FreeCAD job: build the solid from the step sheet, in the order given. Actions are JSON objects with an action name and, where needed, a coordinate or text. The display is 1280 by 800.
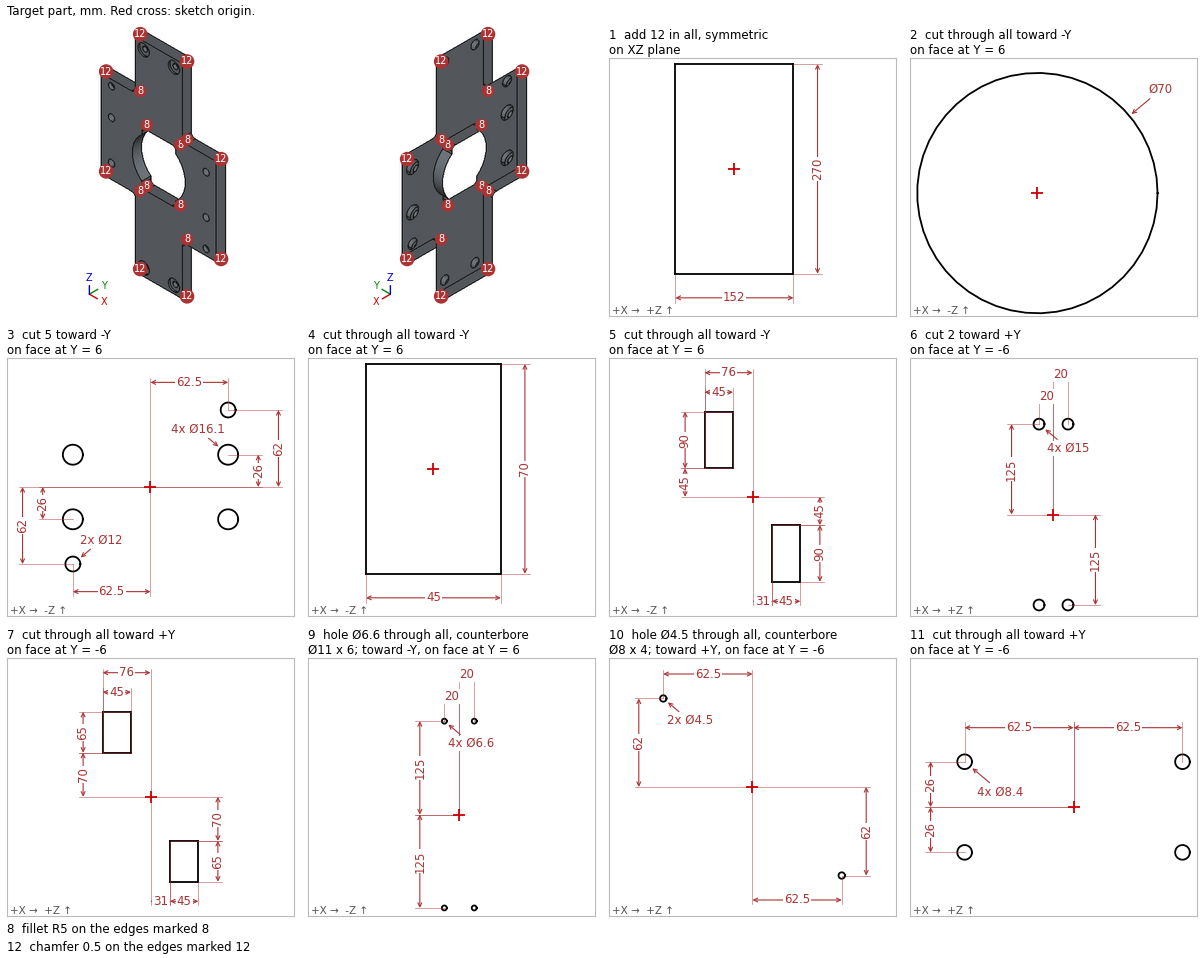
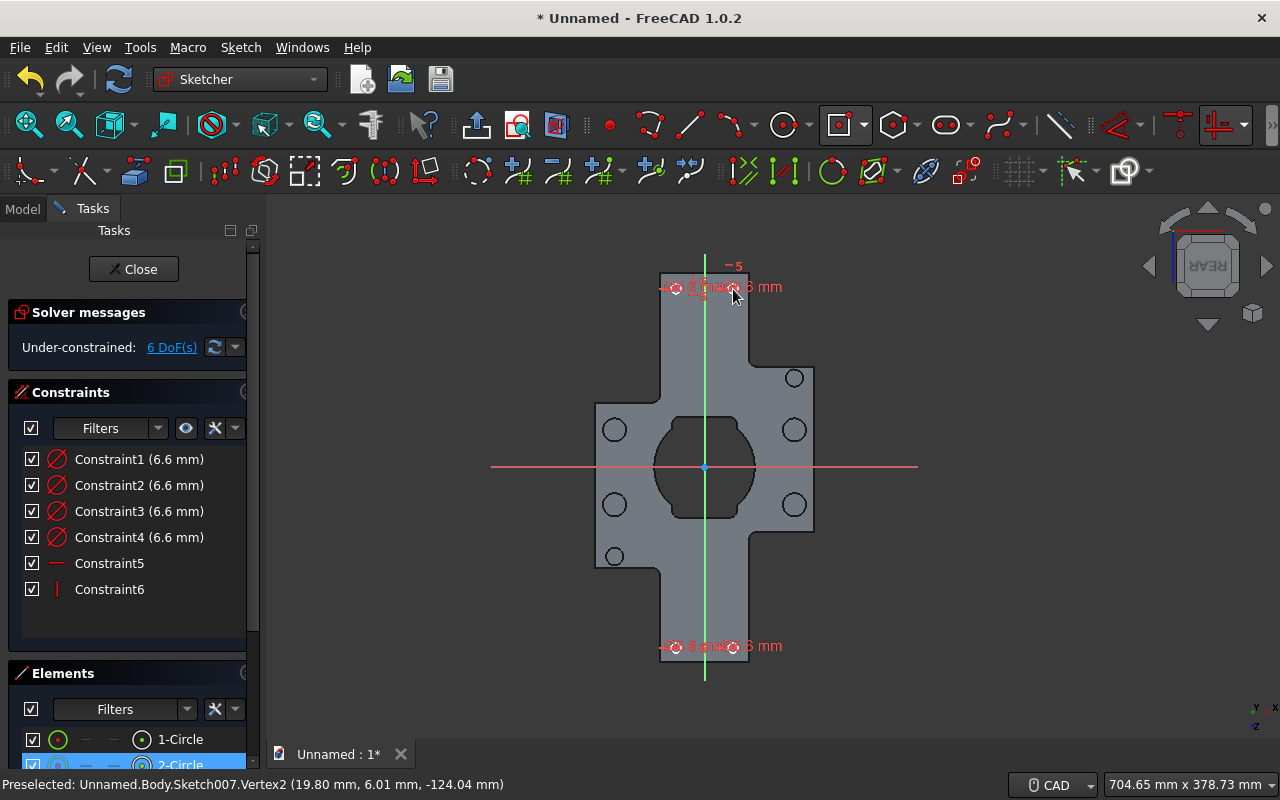
{"action": "left_click", "coordinate": [733, 648]}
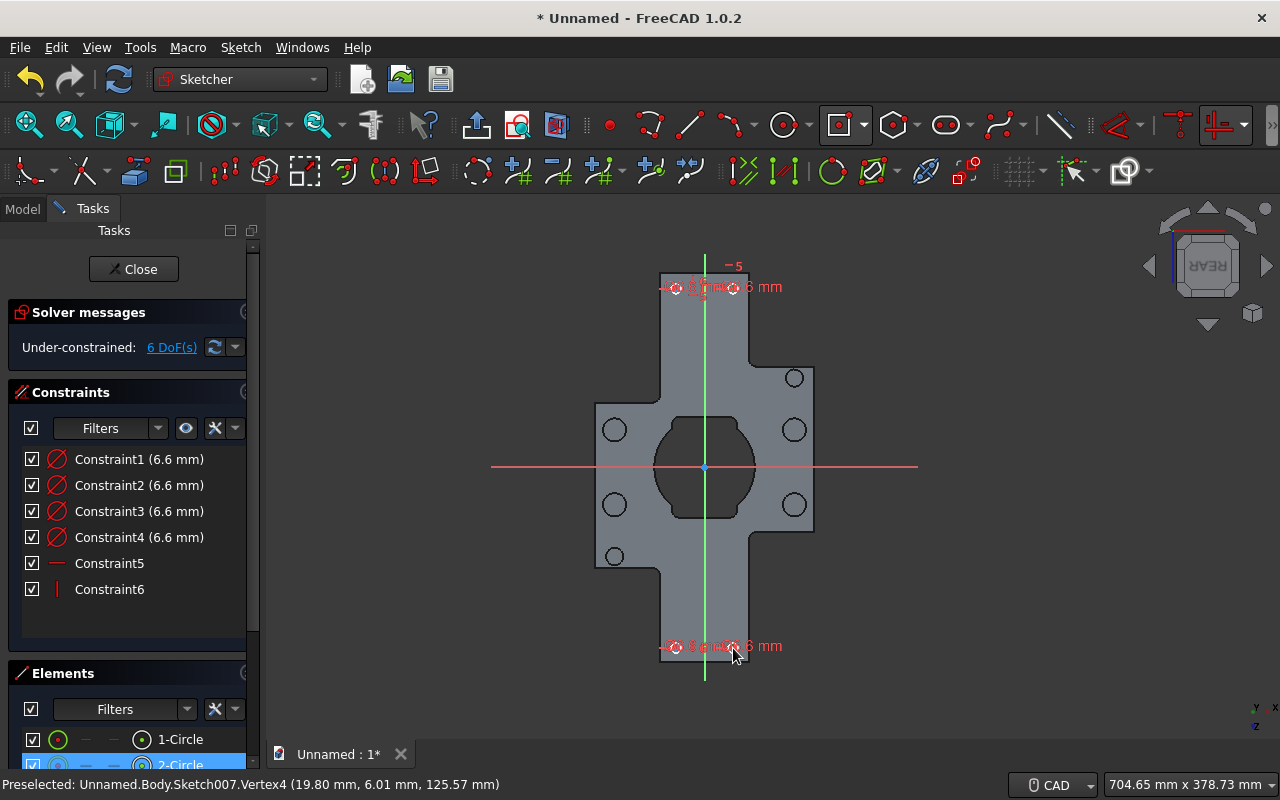
{"action": "key", "text": "v"}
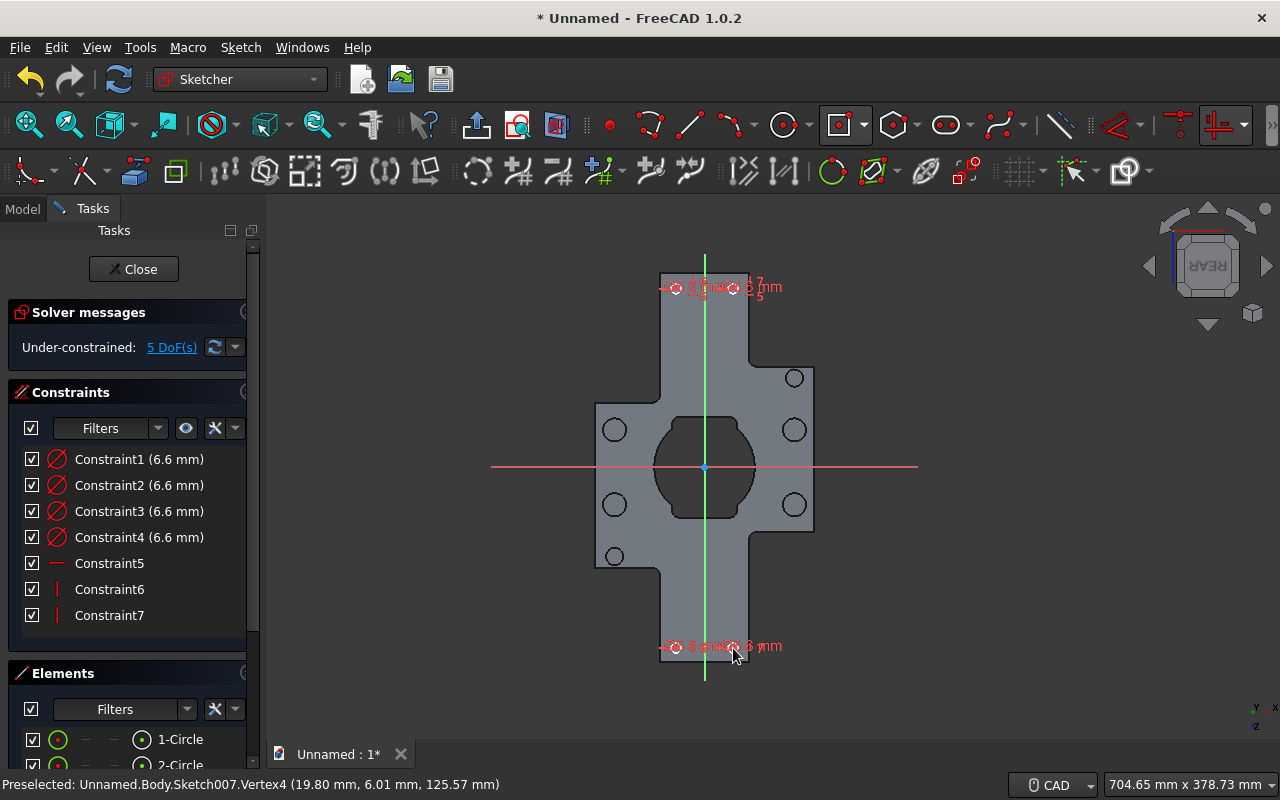
{"action": "left_click", "coordinate": [676, 648]}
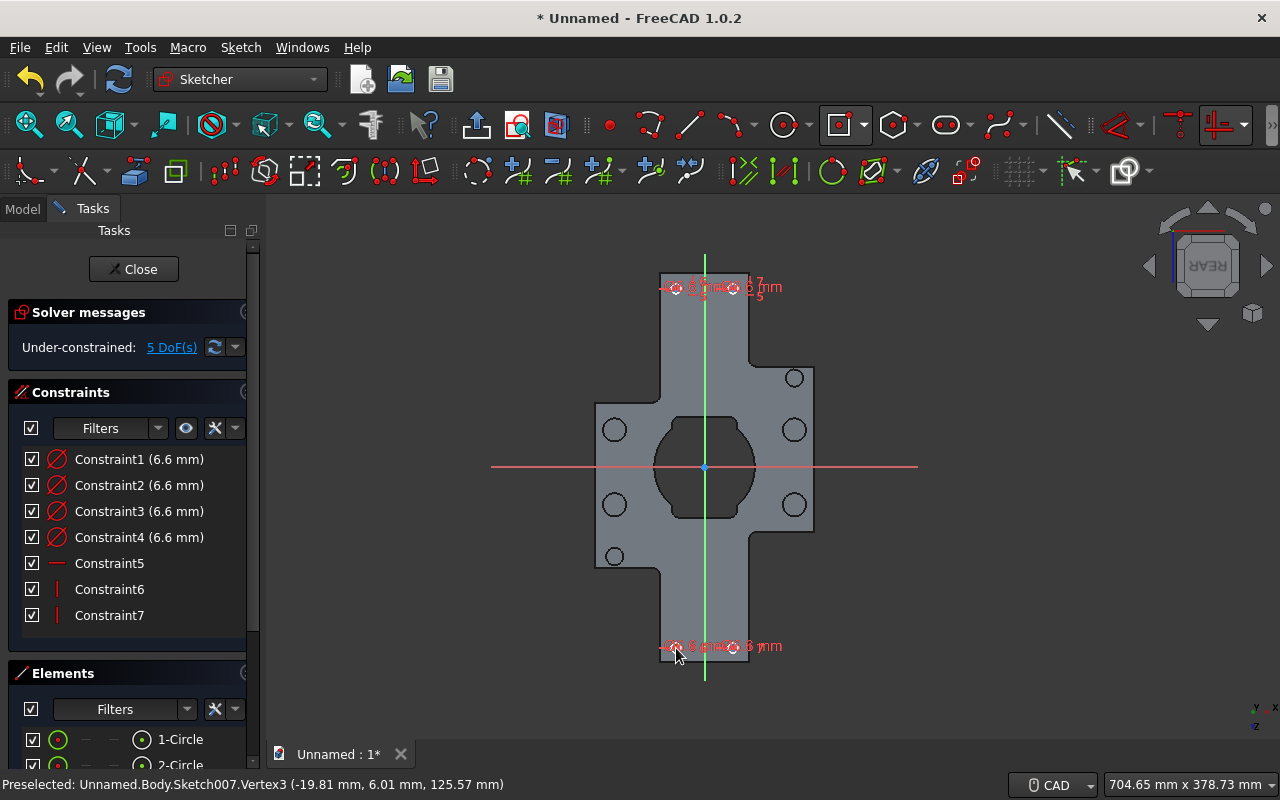
{"action": "left_click", "coordinate": [733, 648]}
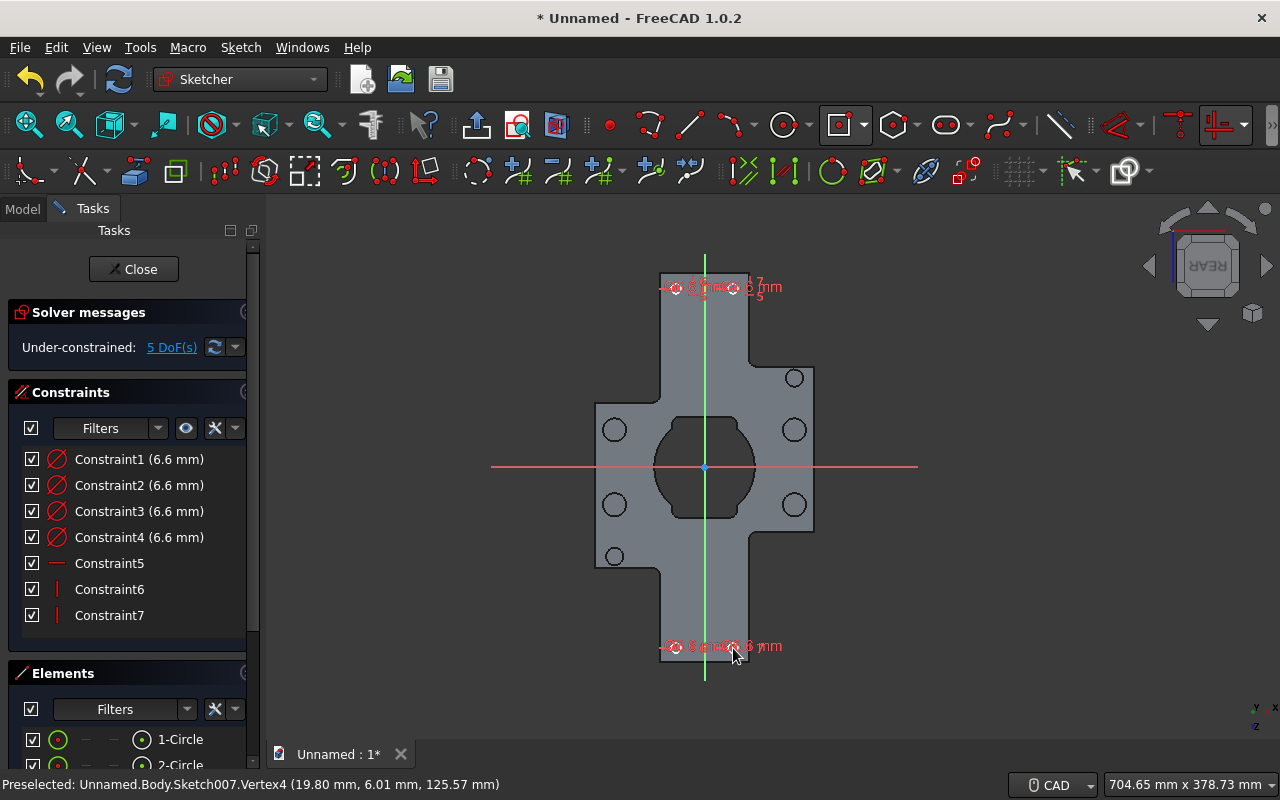
{"action": "key", "text": "h"}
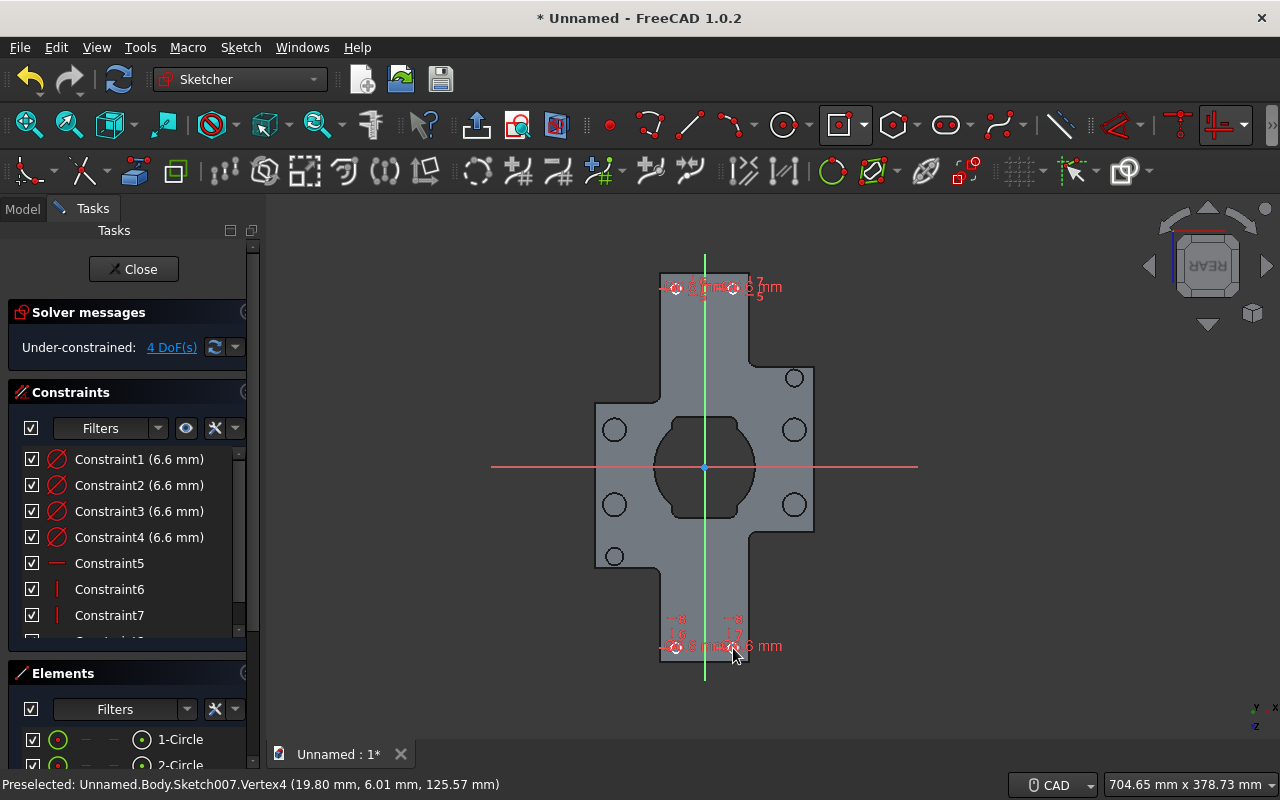
{"action": "key", "text": "d"}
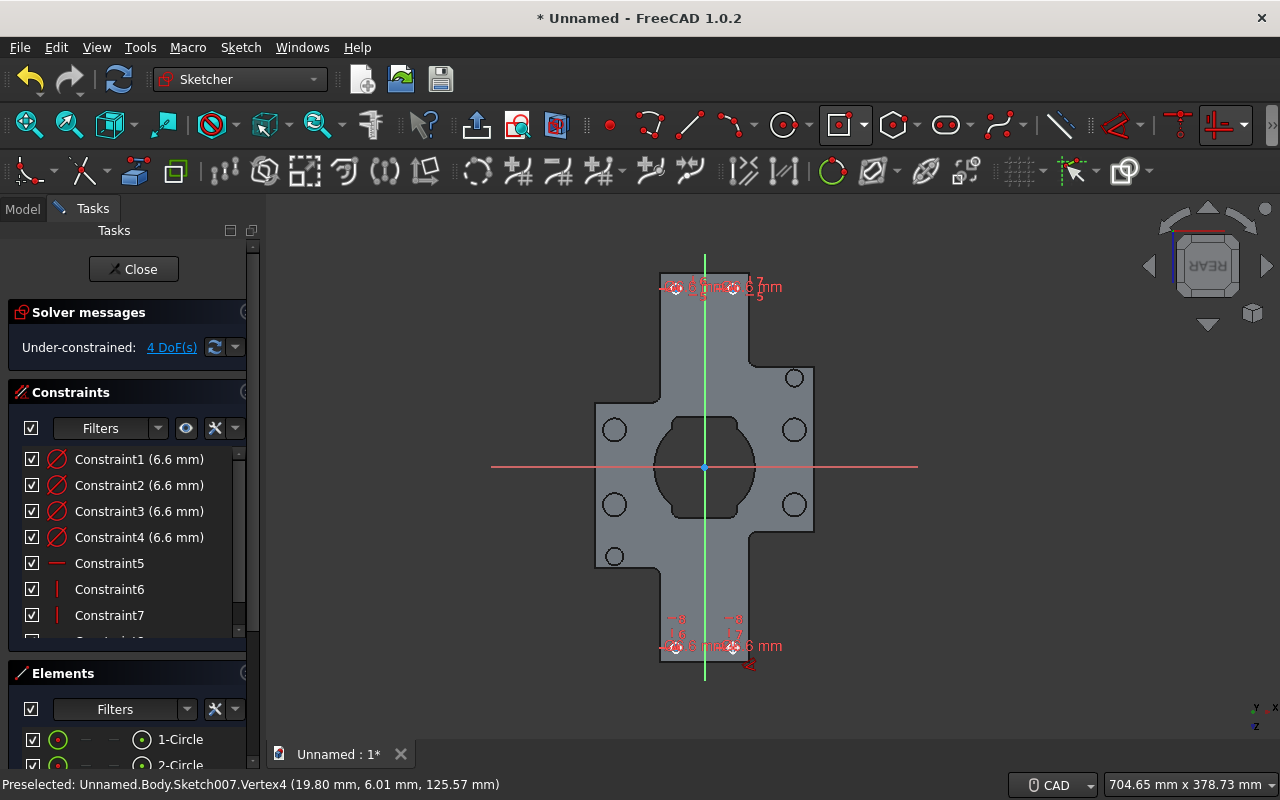
{"action": "scroll", "coordinate": [676, 289], "scroll_direction": "up", "scroll_amount": 2}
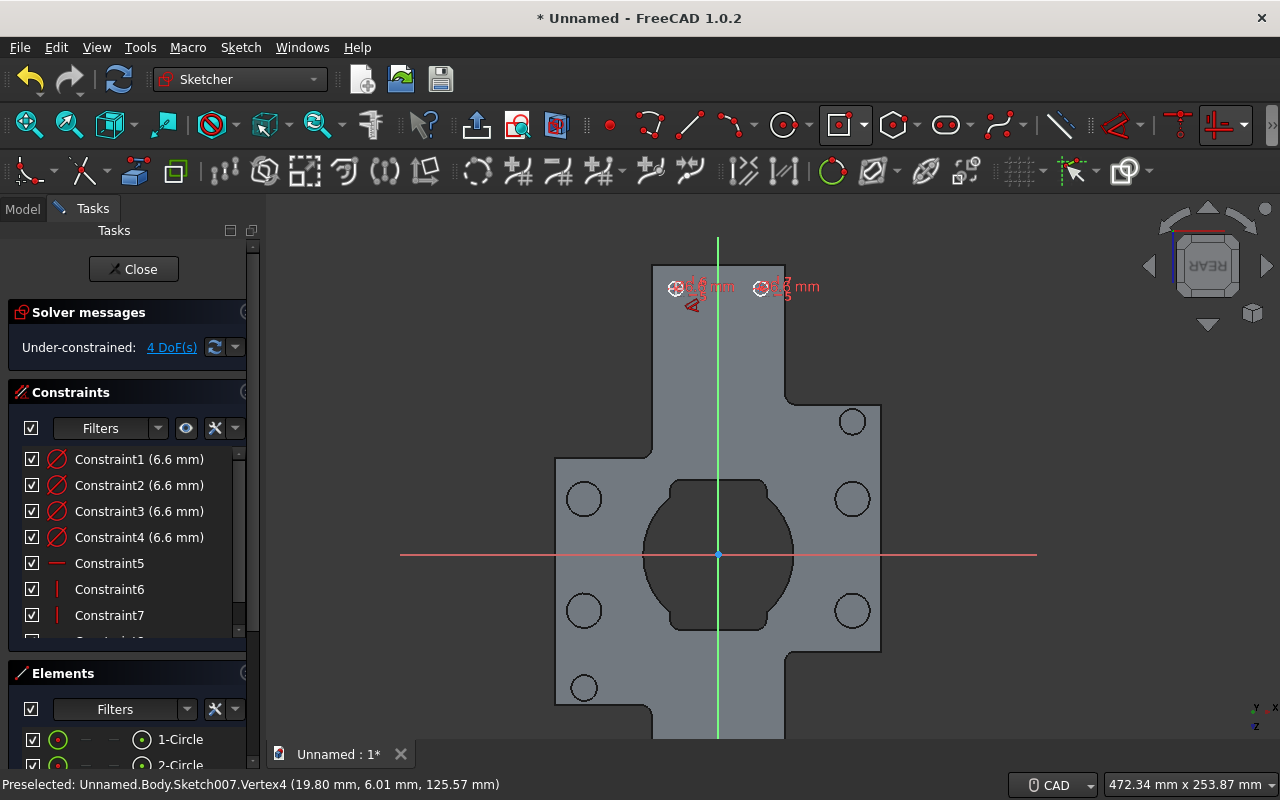
{"action": "left_click", "coordinate": [676, 289]}
{"action": "left_click", "coordinate": [697, 255]}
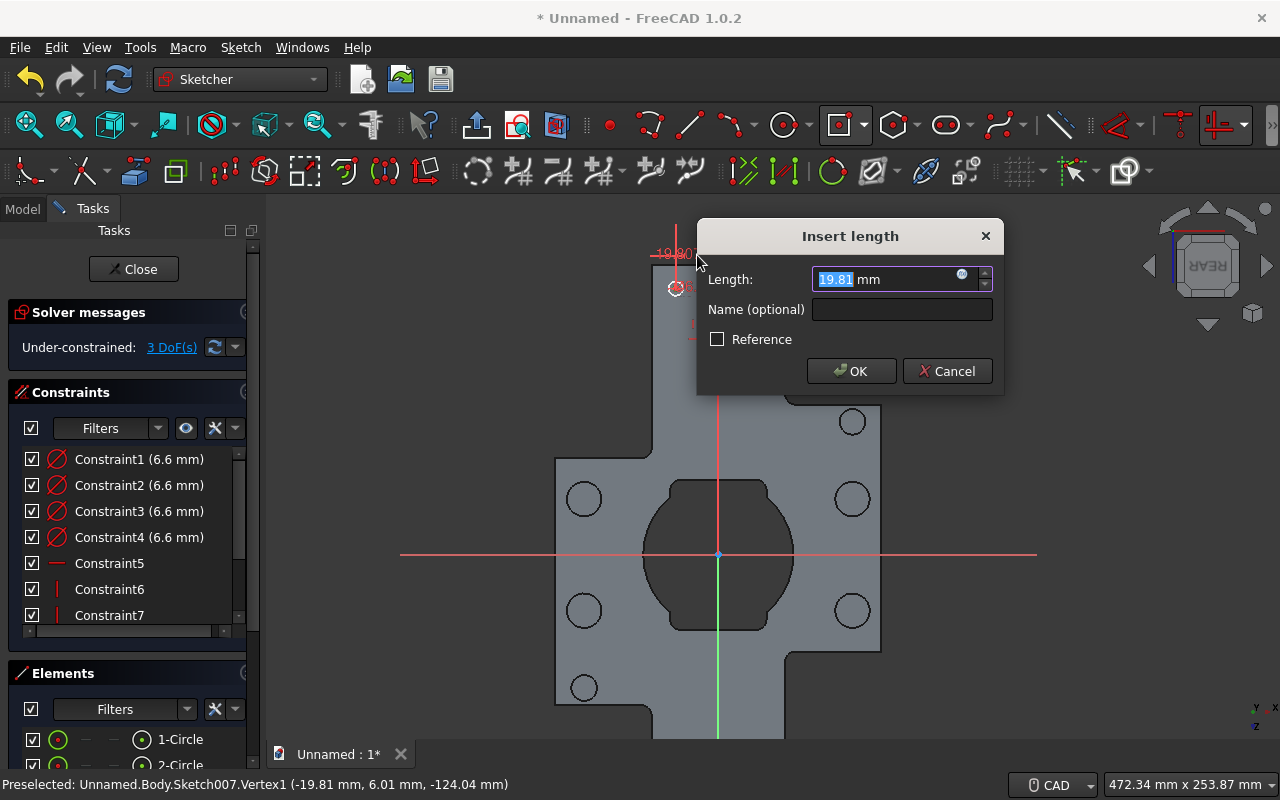
{"action": "type", "text": "20"}
{"action": "key", "text": "Return"}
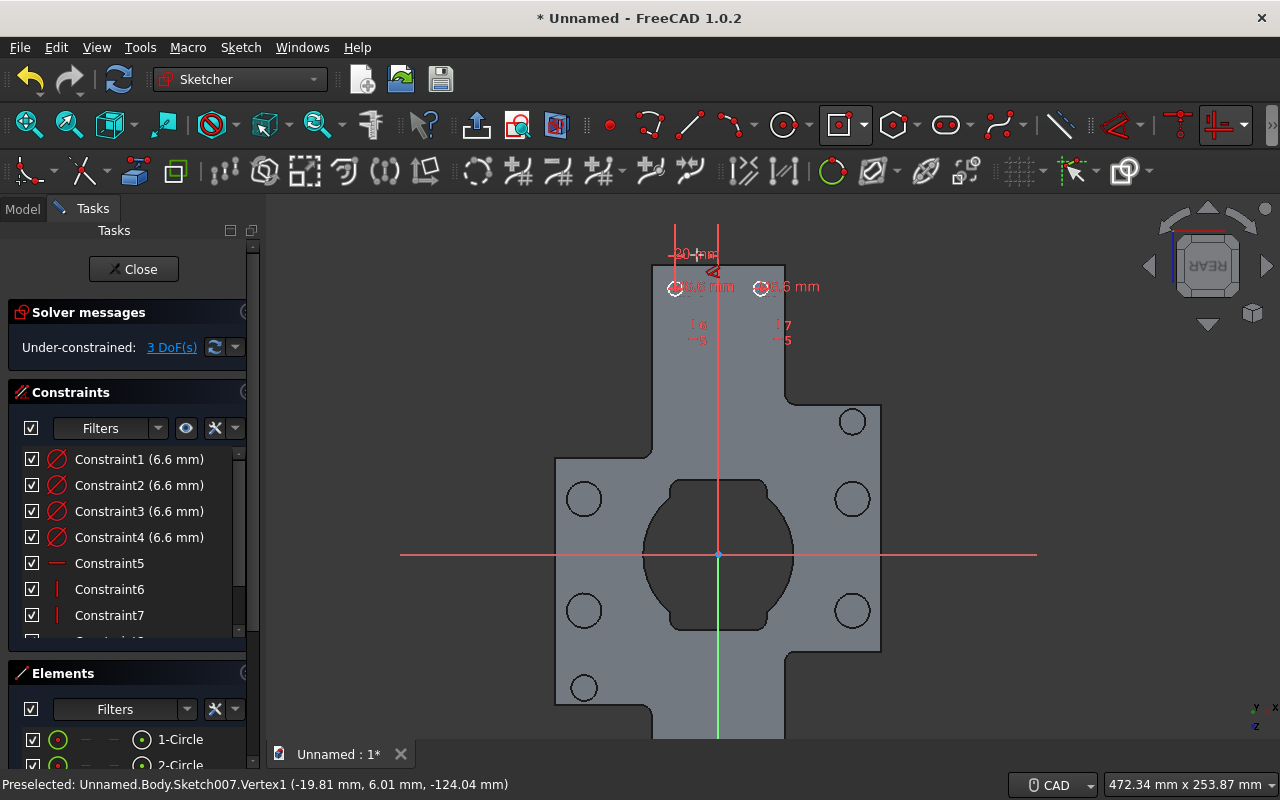
{"action": "left_click", "coordinate": [761, 289]}
{"action": "left_click", "coordinate": [740, 589]}